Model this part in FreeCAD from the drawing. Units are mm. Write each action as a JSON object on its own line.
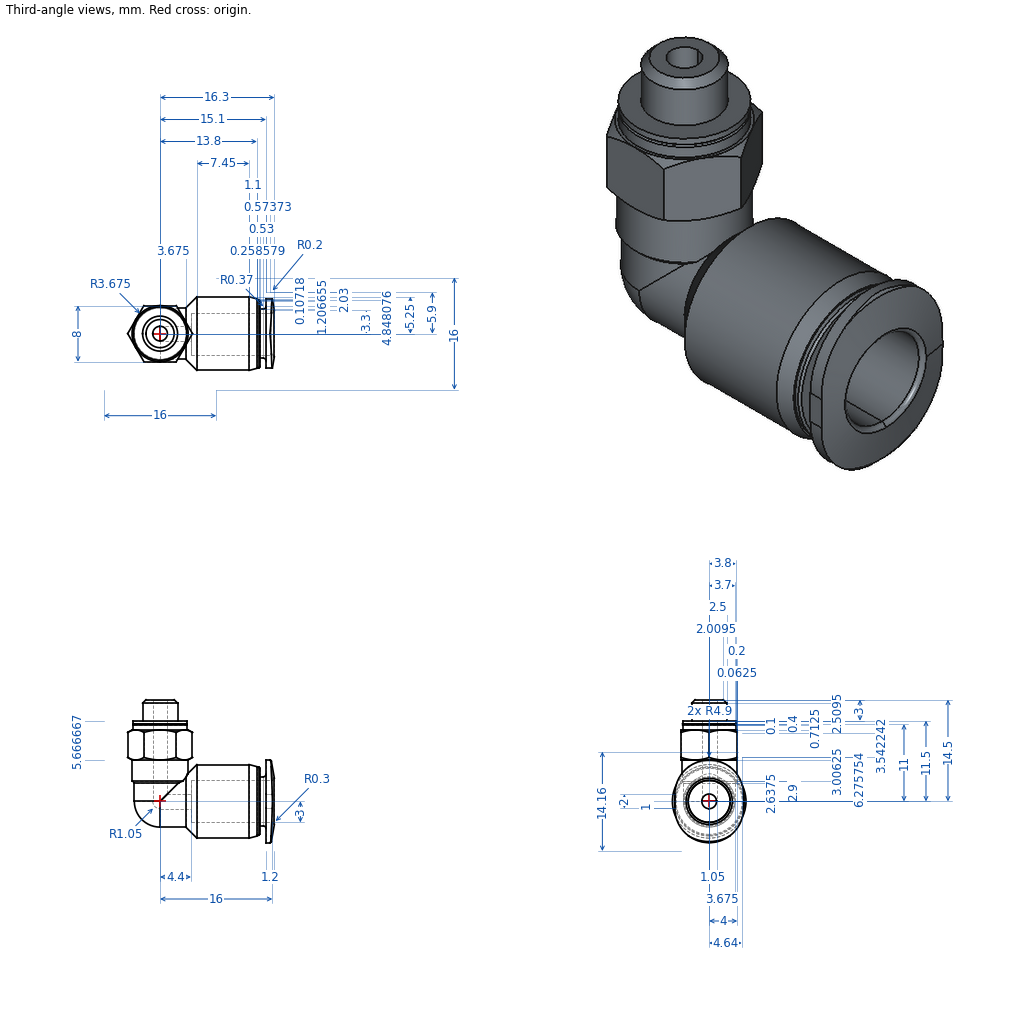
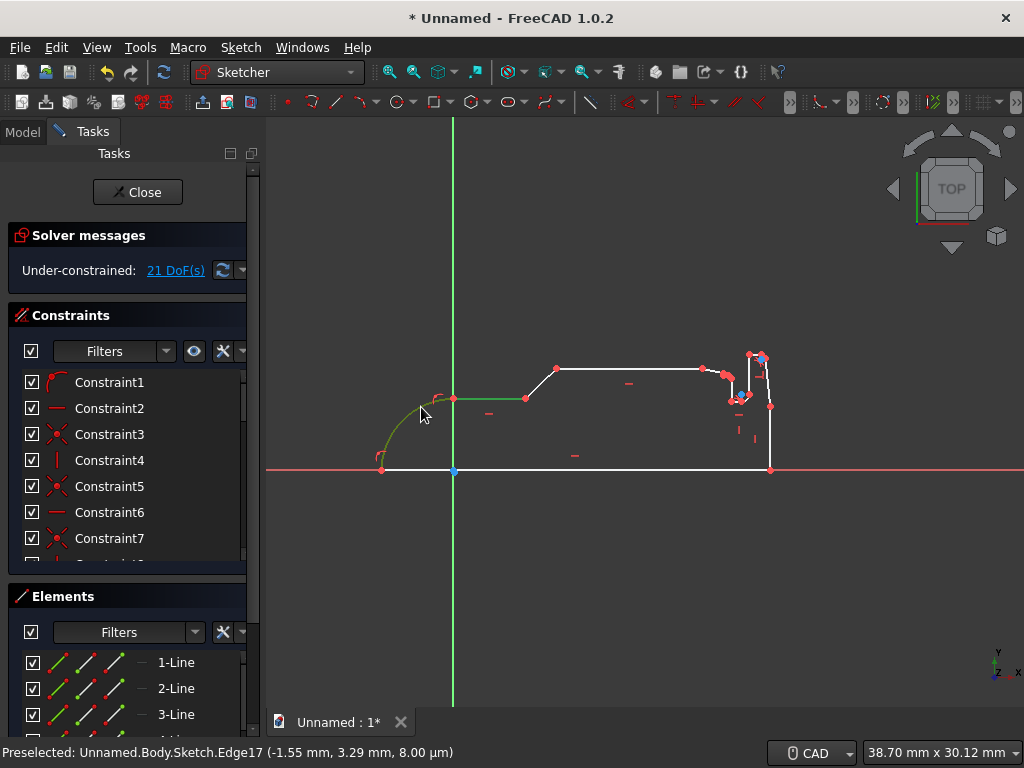
{"action": "key", "text": "t"}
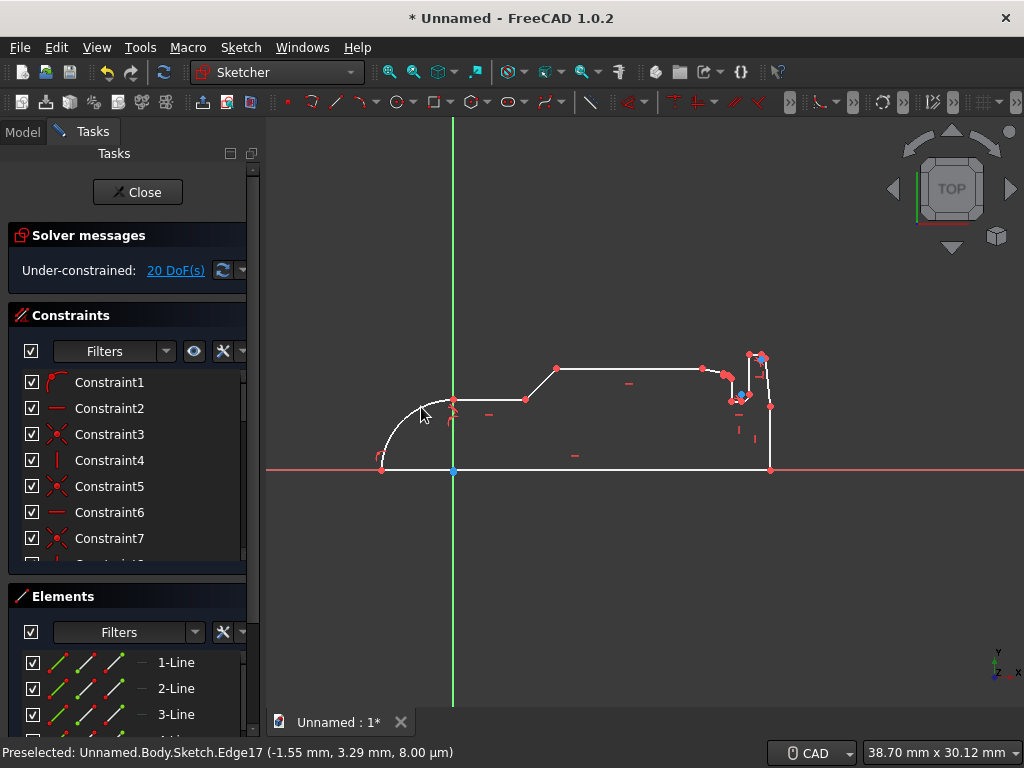
{"action": "left_click", "coordinate": [453, 472]}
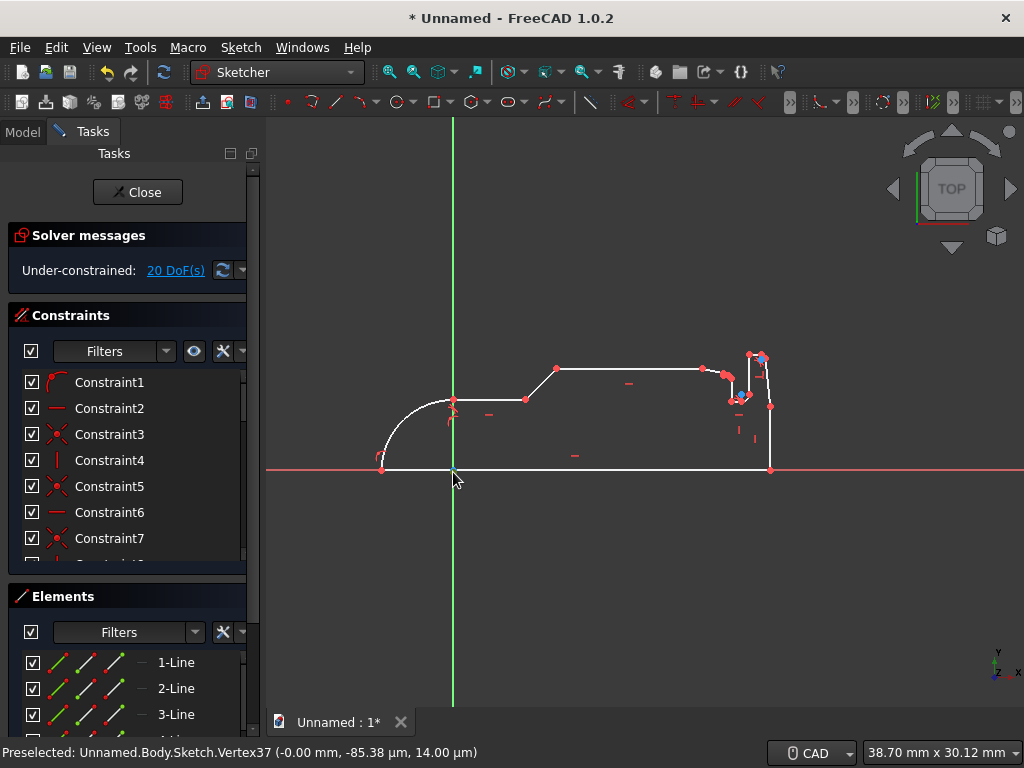
{"action": "left_click", "coordinate": [334, 470]}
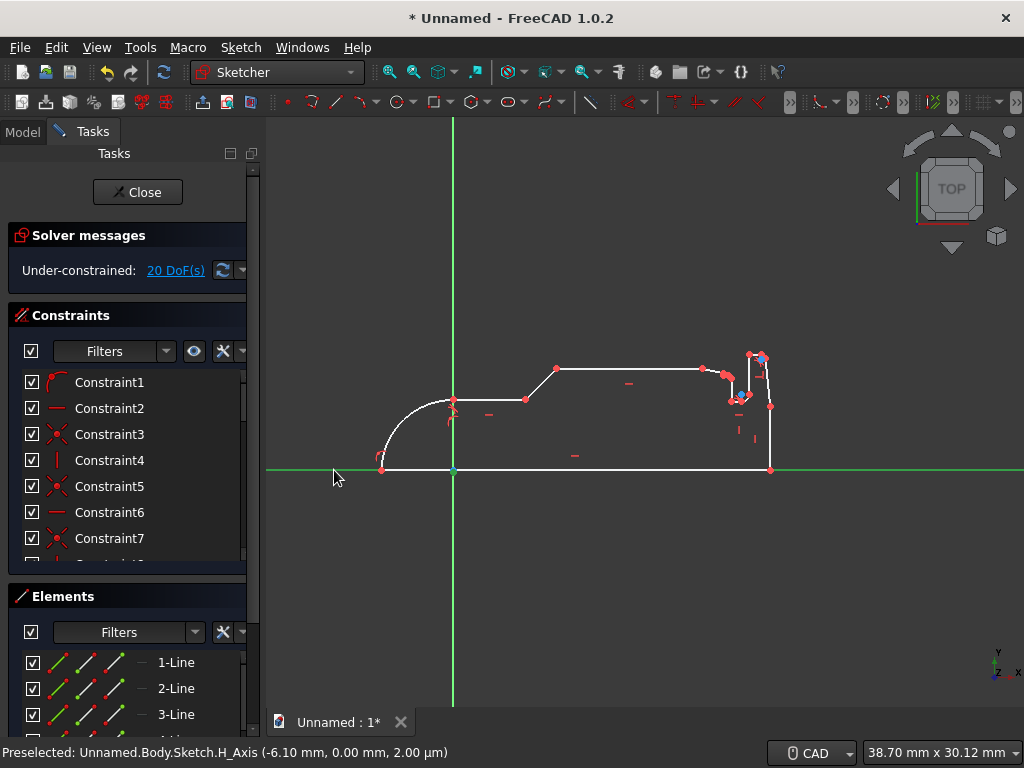
{"action": "left_click", "coordinate": [674, 102]}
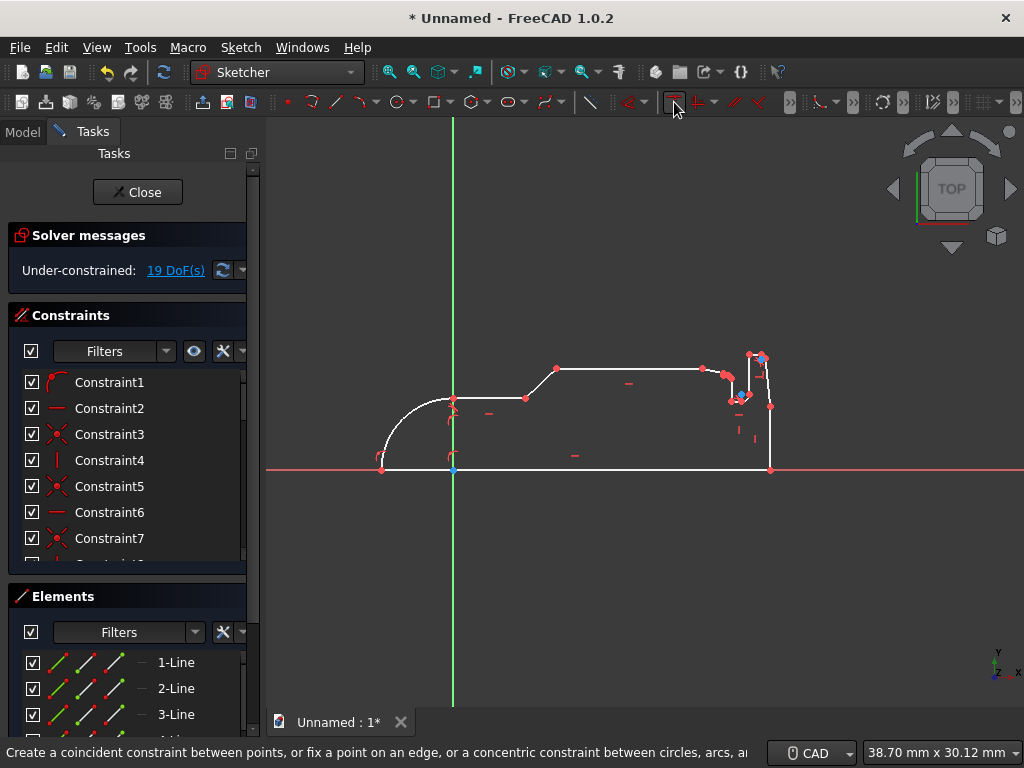
{"action": "left_click", "coordinate": [628, 102]}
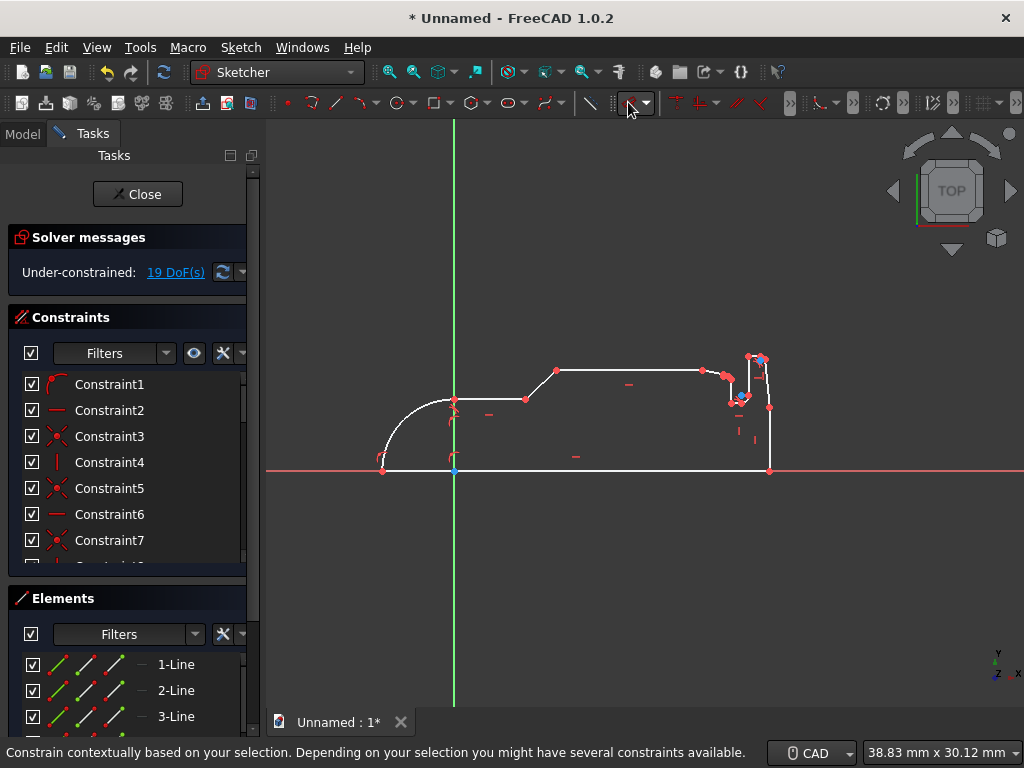
{"action": "scroll", "coordinate": [764, 357], "scroll_direction": "up", "scroll_amount": 12}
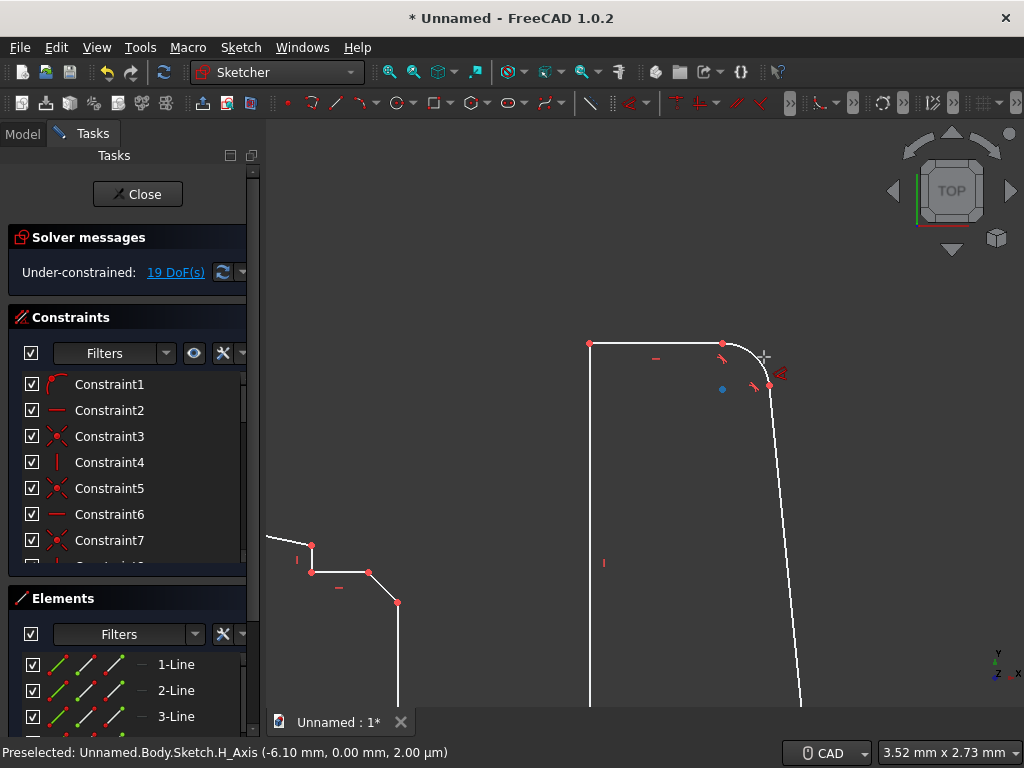
{"action": "left_click", "coordinate": [754, 355]}
{"action": "left_click", "coordinate": [775, 331]}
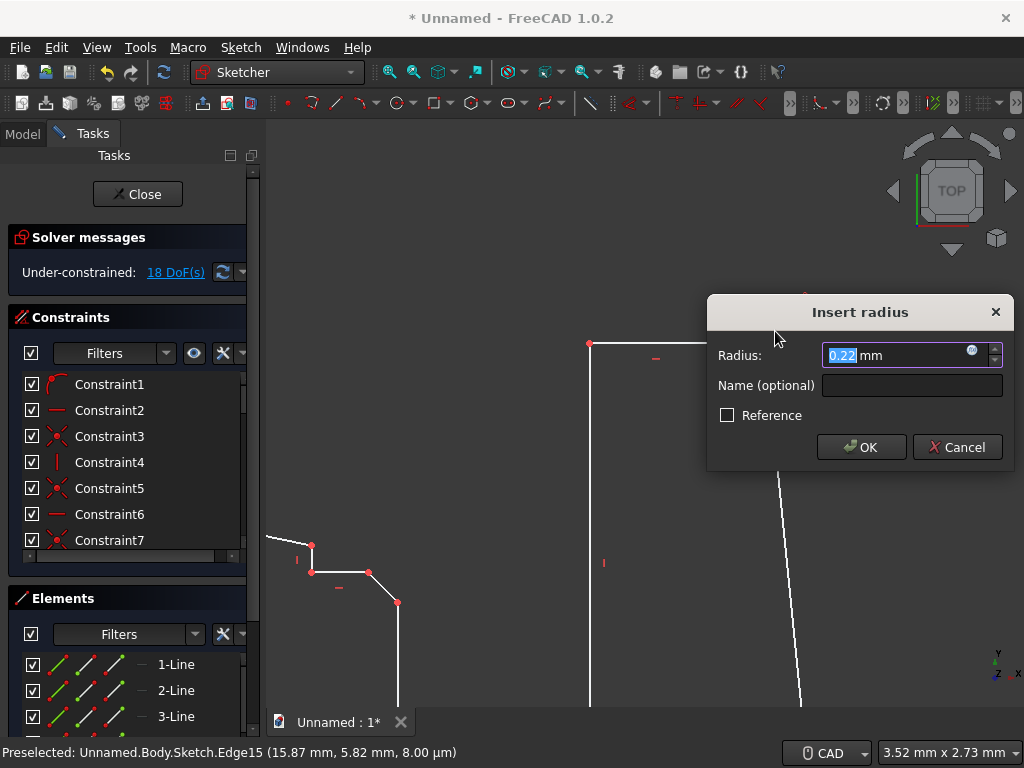
{"action": "type", "text": "0.2"}
{"action": "key", "text": "Return"}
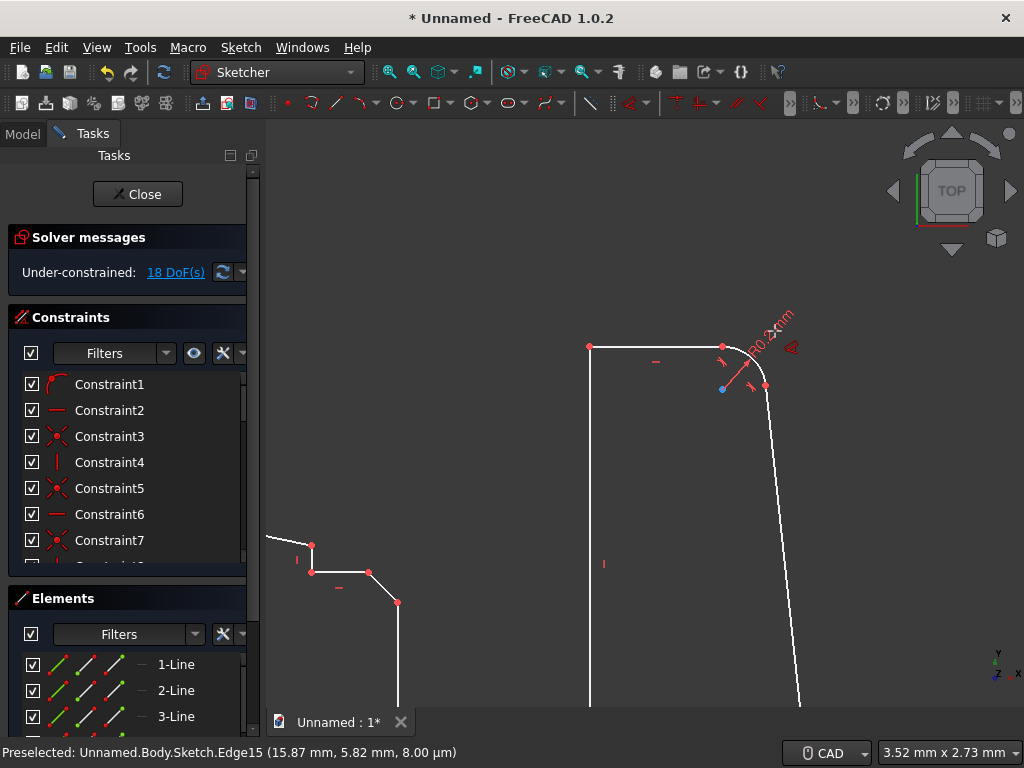
{"action": "scroll", "coordinate": [764, 357], "scroll_direction": "down", "scroll_amount": 12}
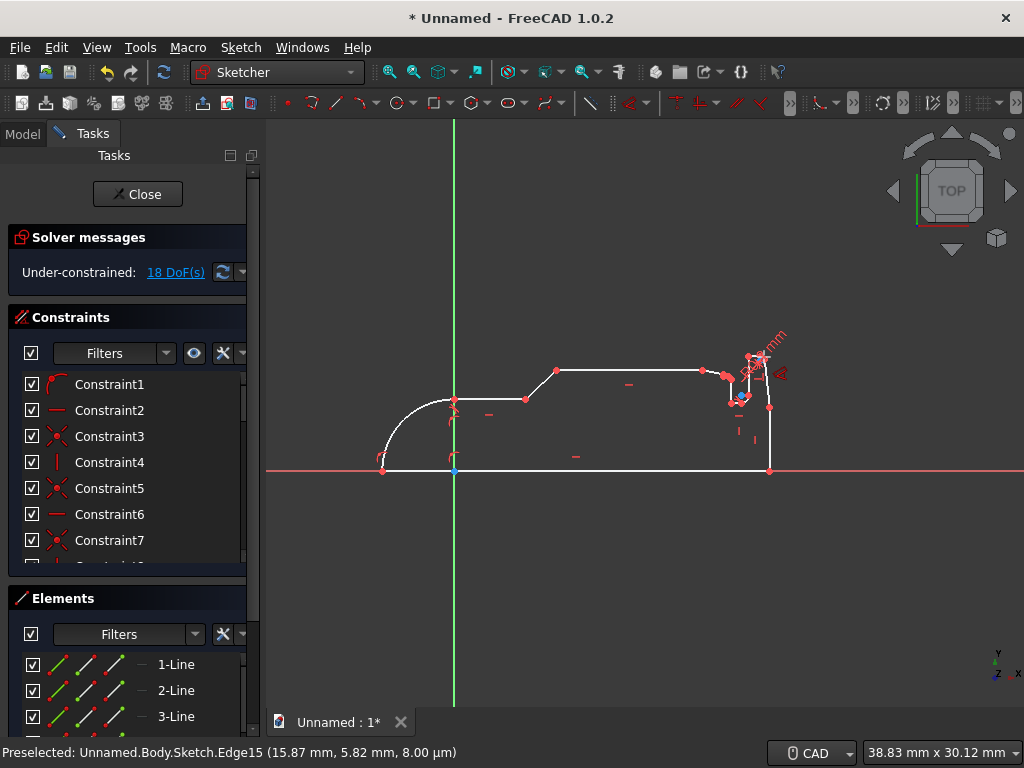
{"action": "scroll", "coordinate": [745, 402], "scroll_direction": "up", "scroll_amount": 9}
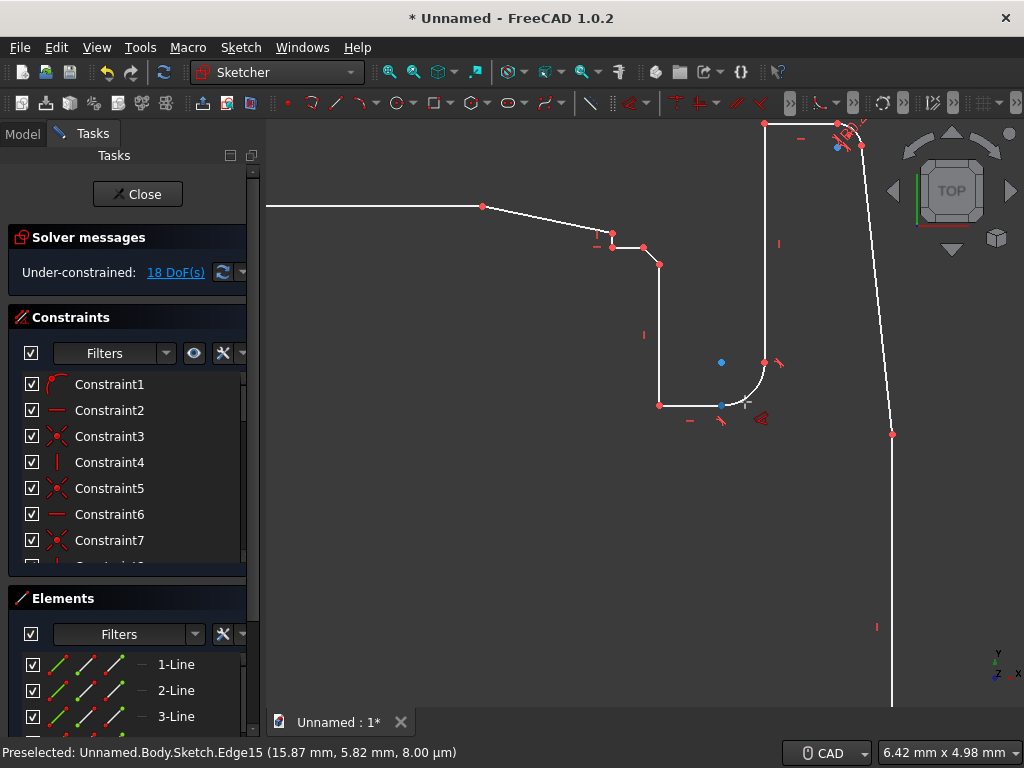
{"action": "left_click", "coordinate": [741, 401]}
{"action": "left_click", "coordinate": [756, 429]}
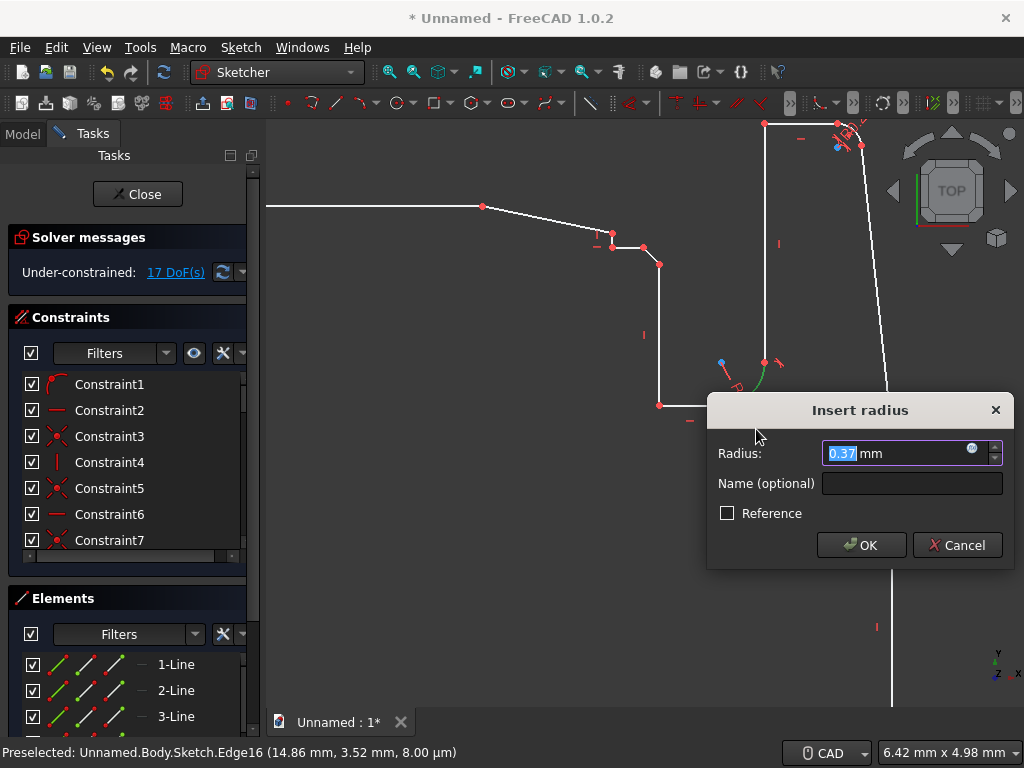
{"action": "type", "text": "0.37"}
{"action": "key", "text": "Return"}